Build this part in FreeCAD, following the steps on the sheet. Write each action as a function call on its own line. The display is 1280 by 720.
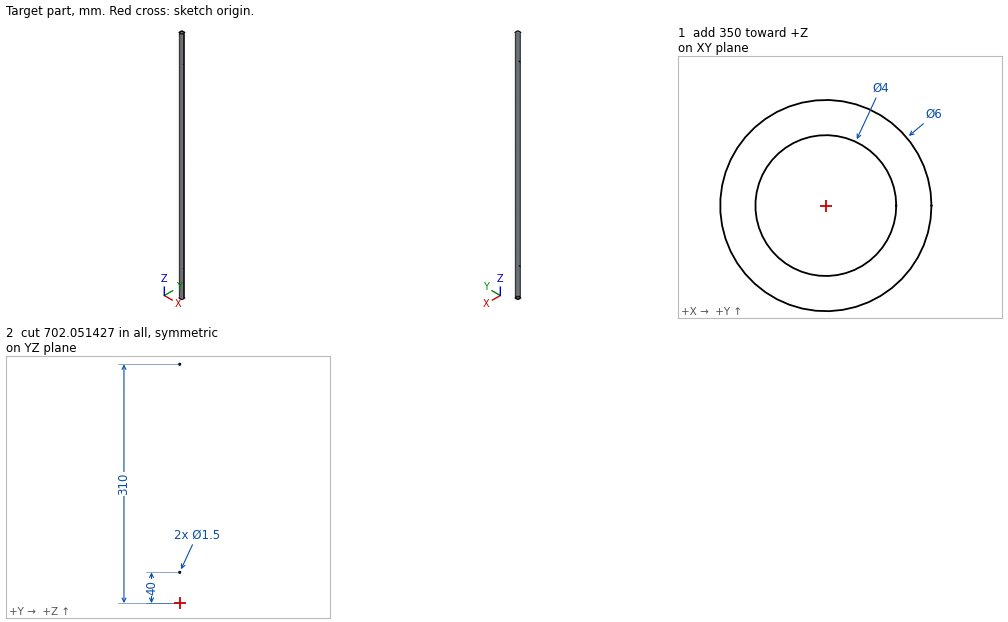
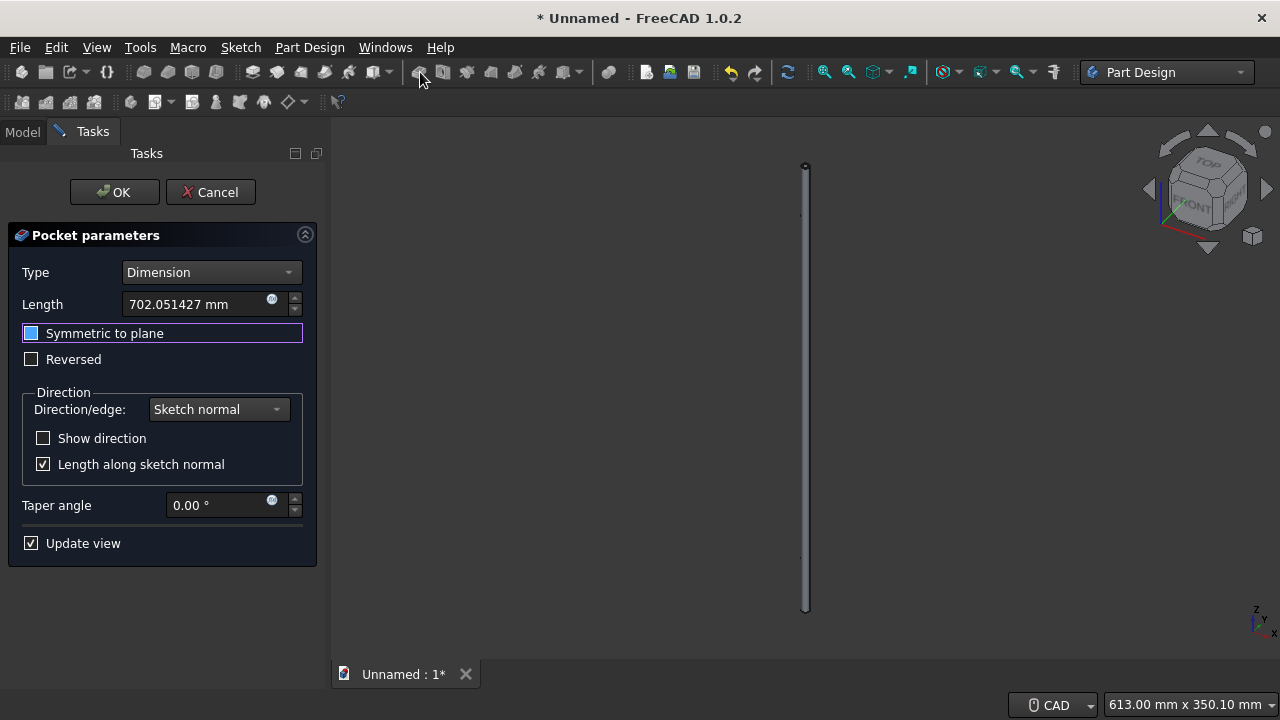
click(30, 333)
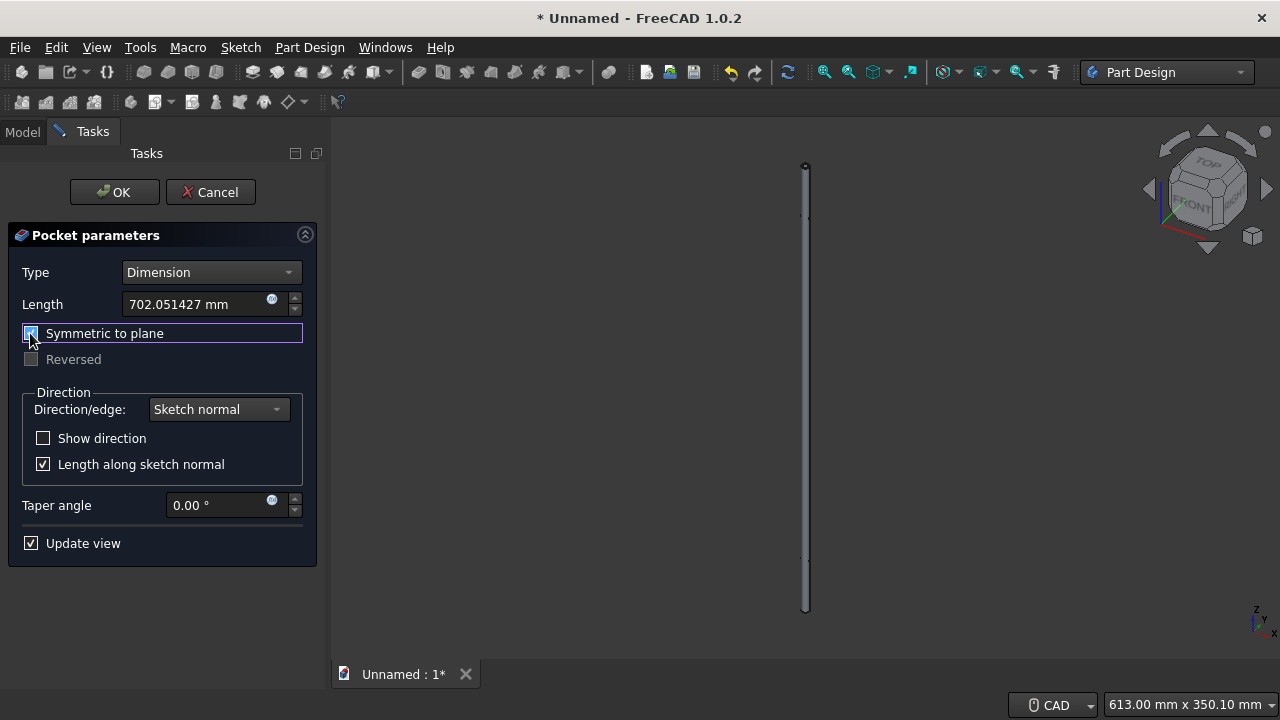
click(115, 192)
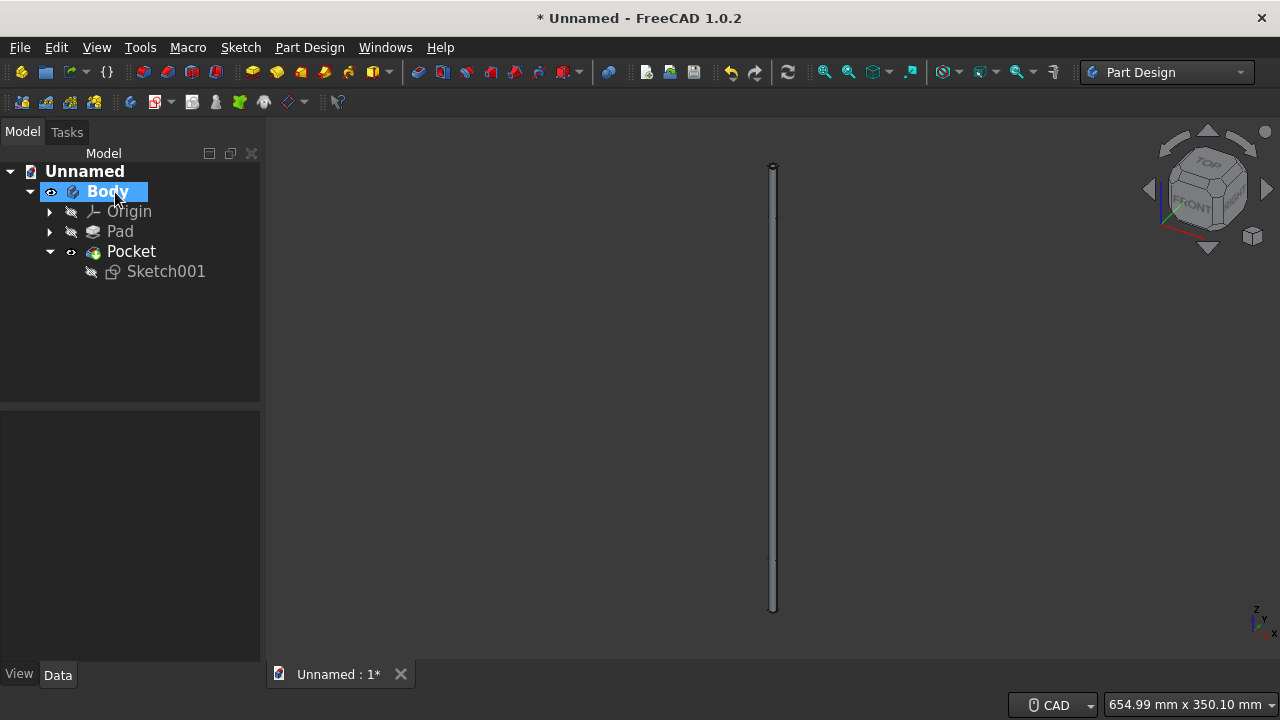
key(0)